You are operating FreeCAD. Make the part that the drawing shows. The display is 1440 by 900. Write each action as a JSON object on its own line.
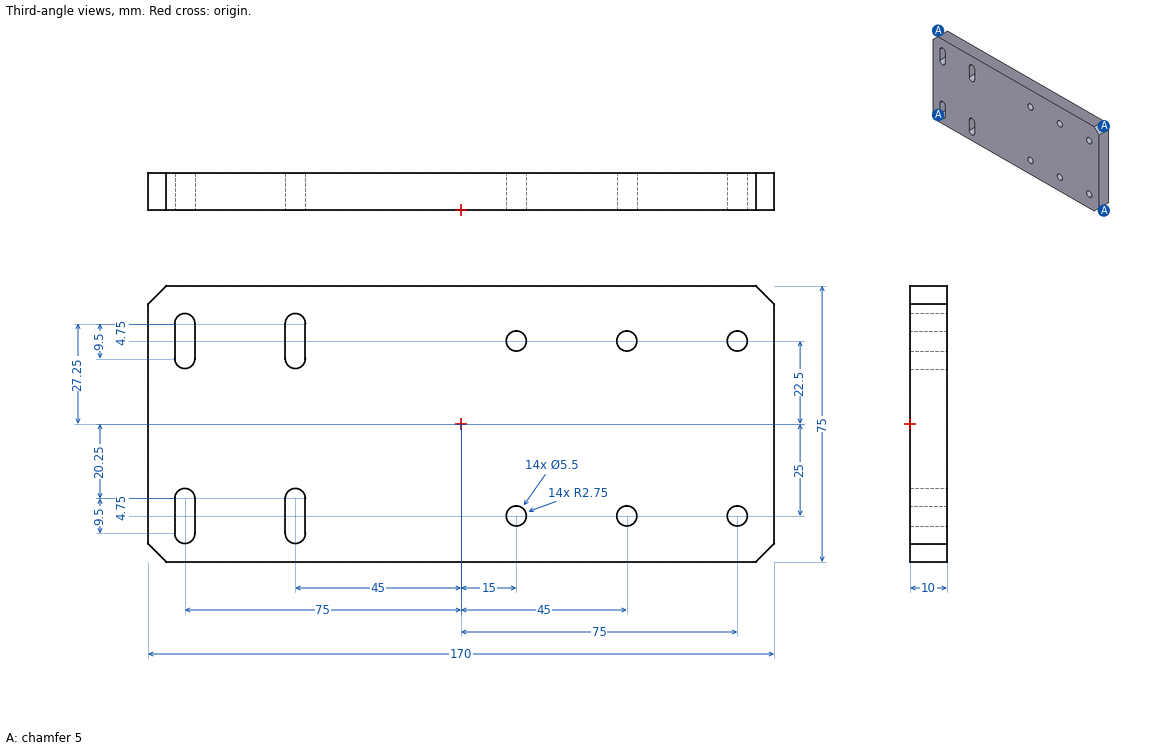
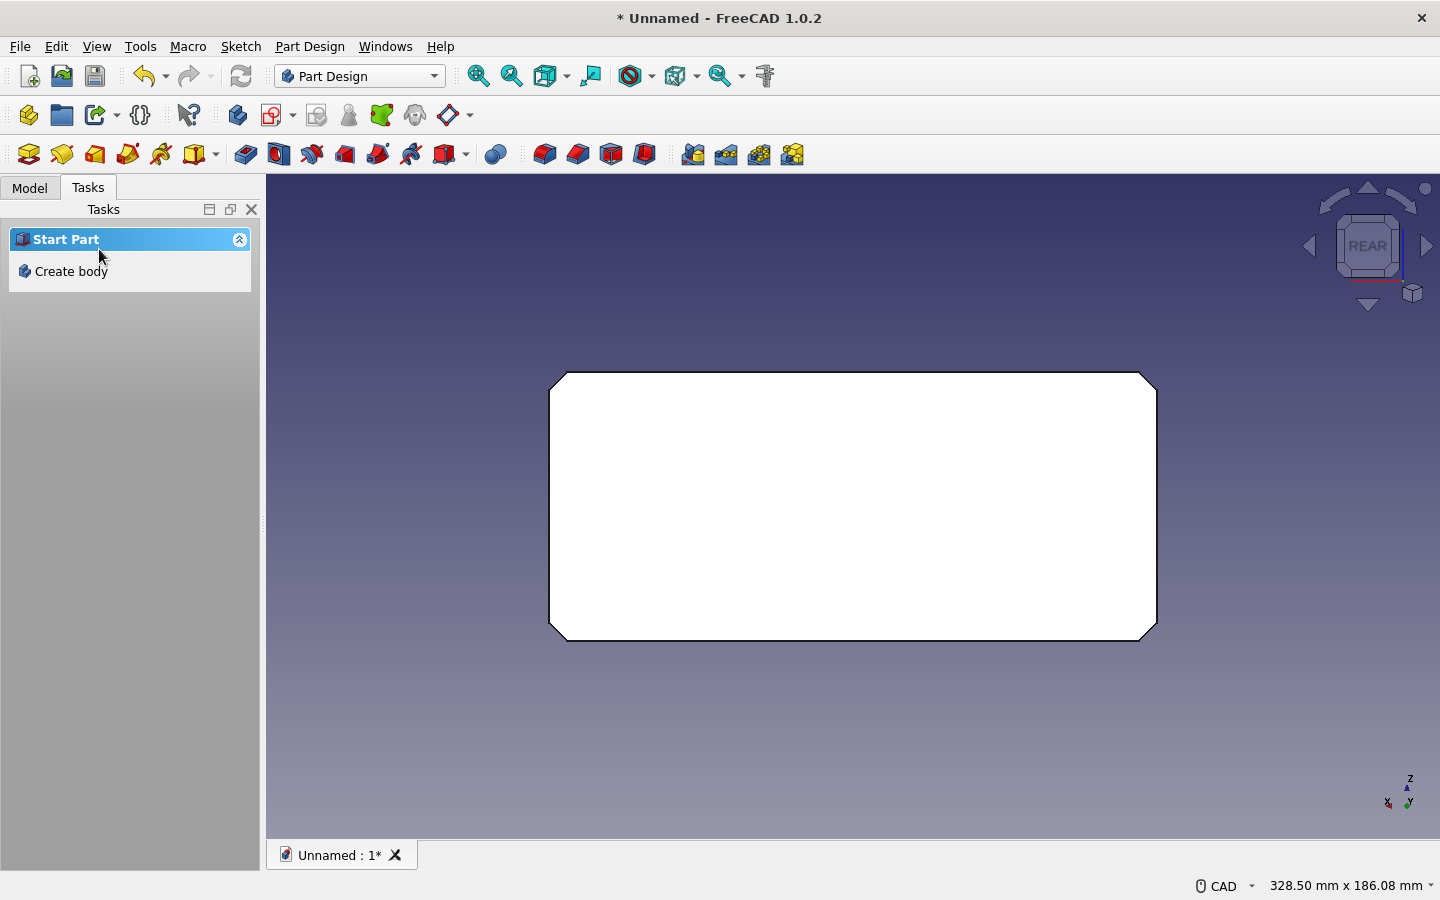
{"action": "left_click", "coordinate": [766, 506]}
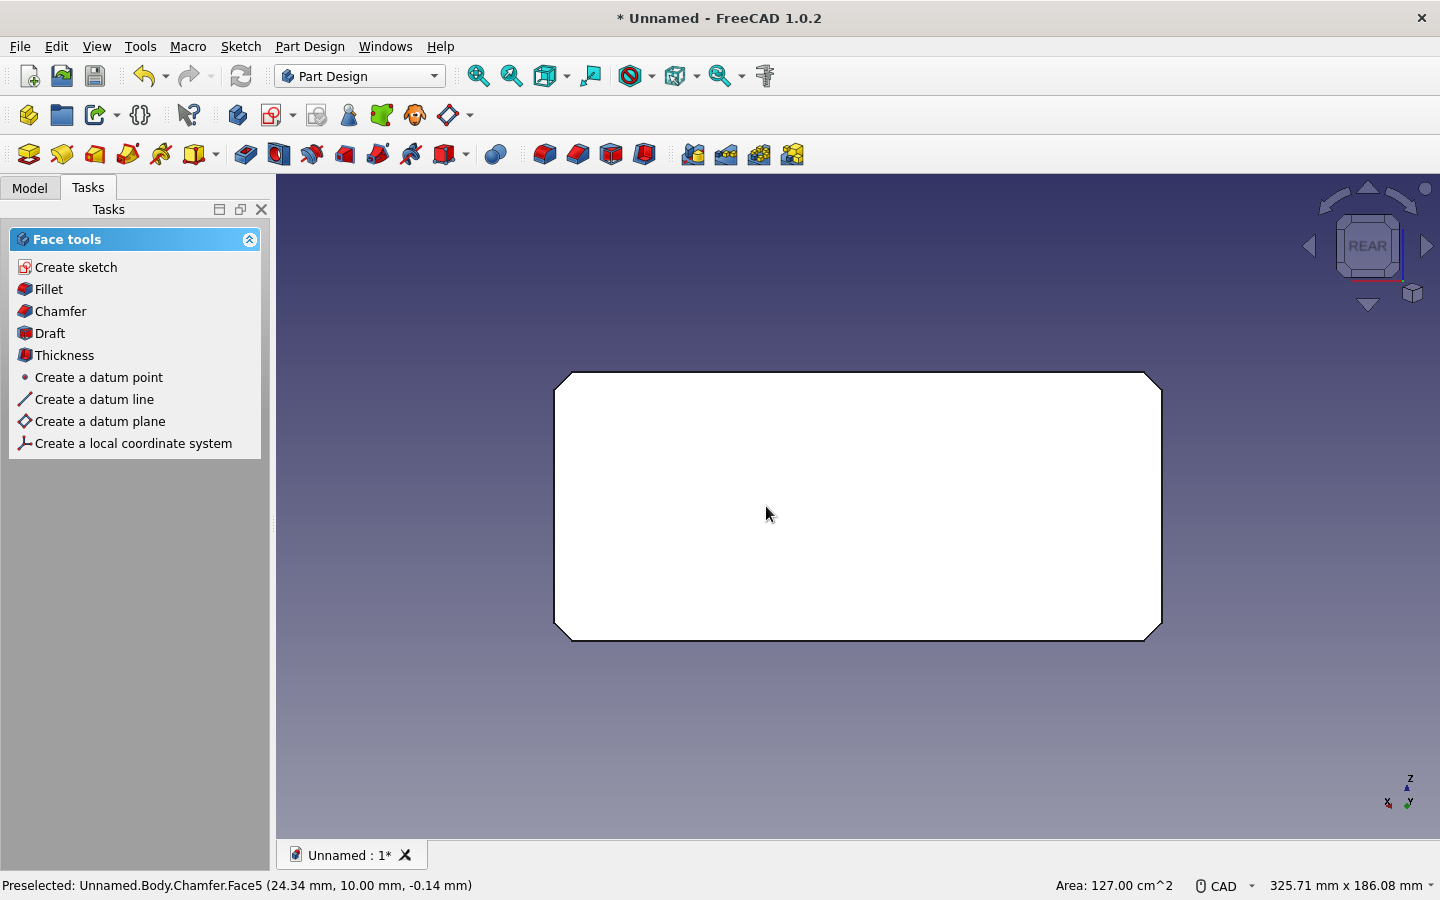
{"action": "left_click", "coordinate": [270, 116]}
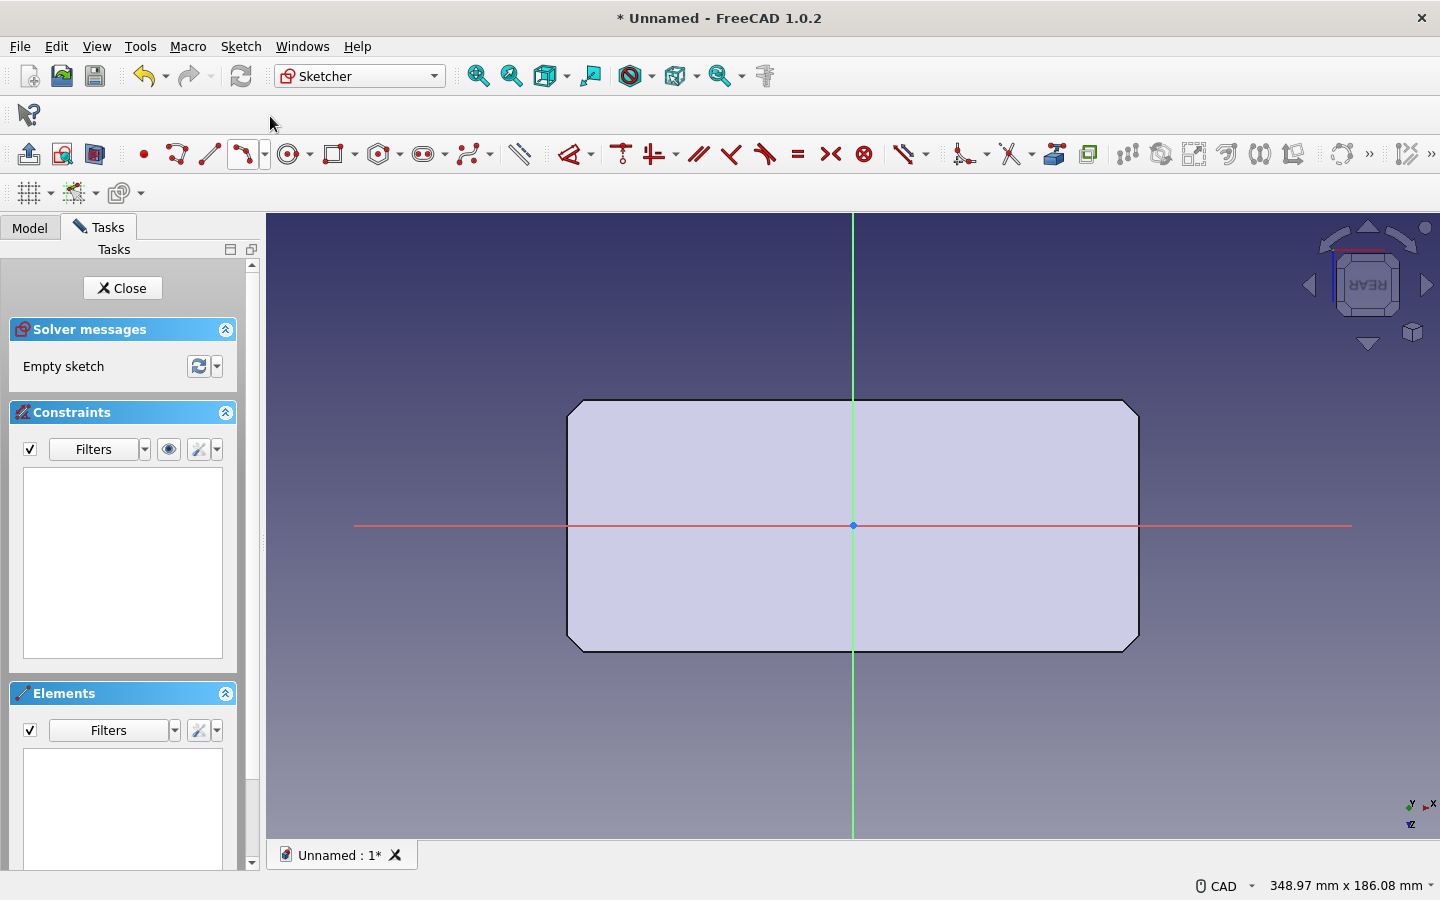
{"action": "key", "text": "g s"}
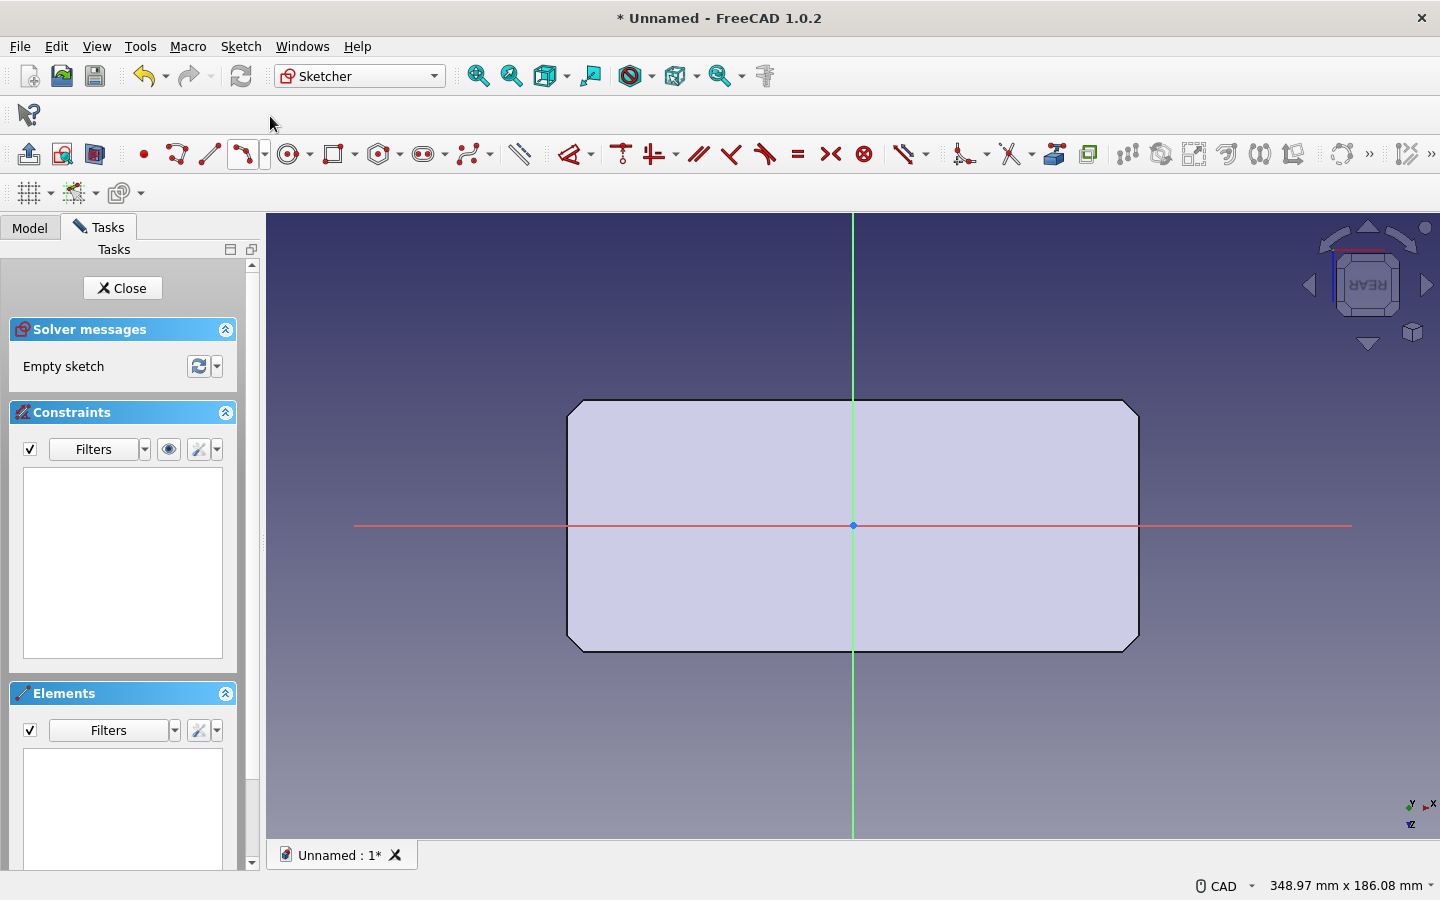
{"action": "scroll", "coordinate": [601, 458], "scroll_direction": "up", "scroll_amount": 5}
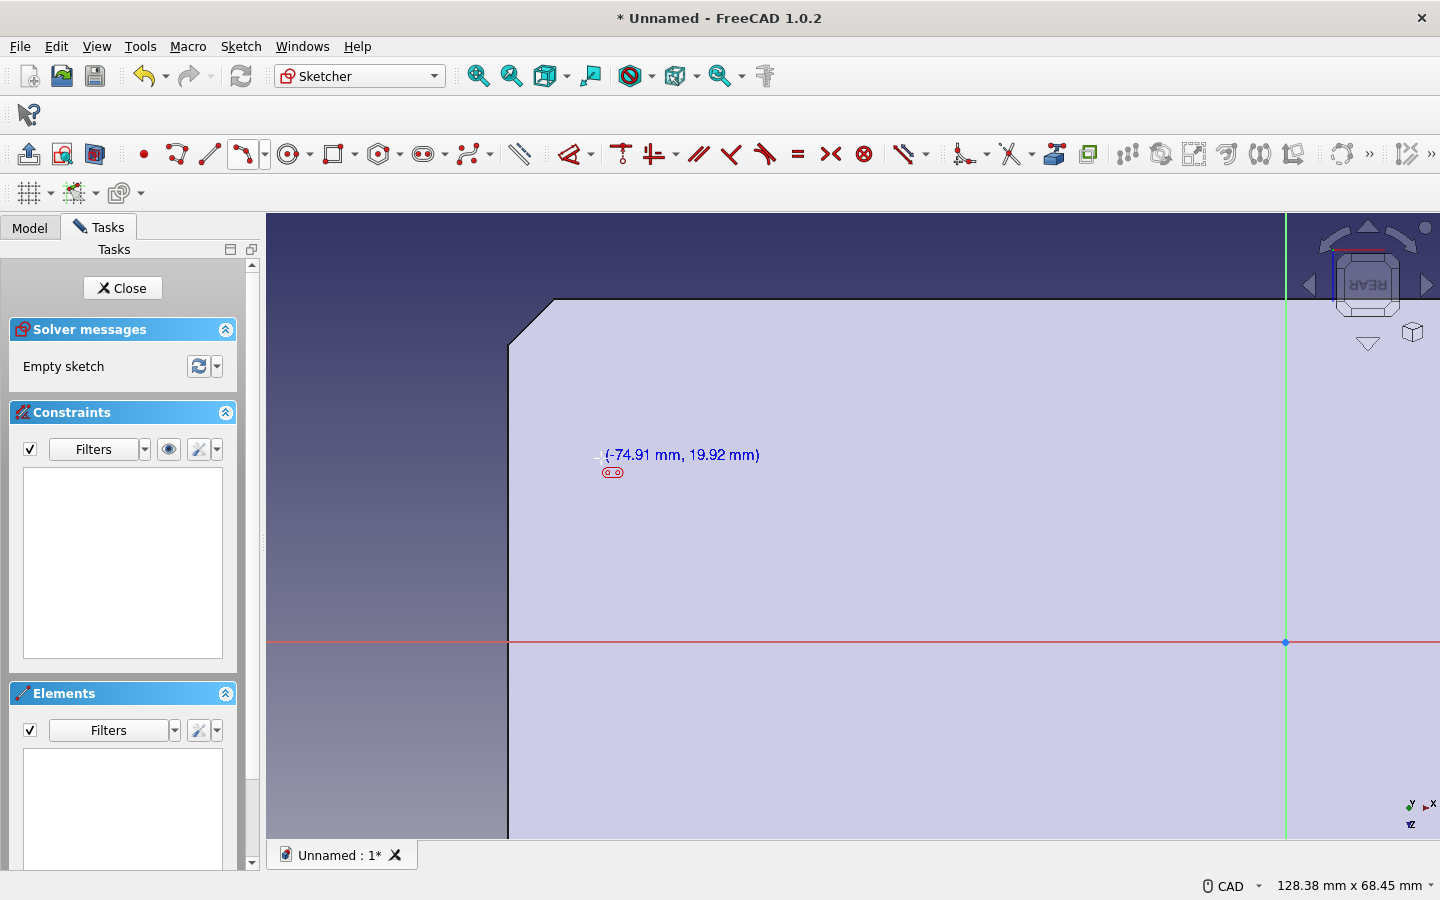
{"action": "left_click", "coordinate": [600, 457]}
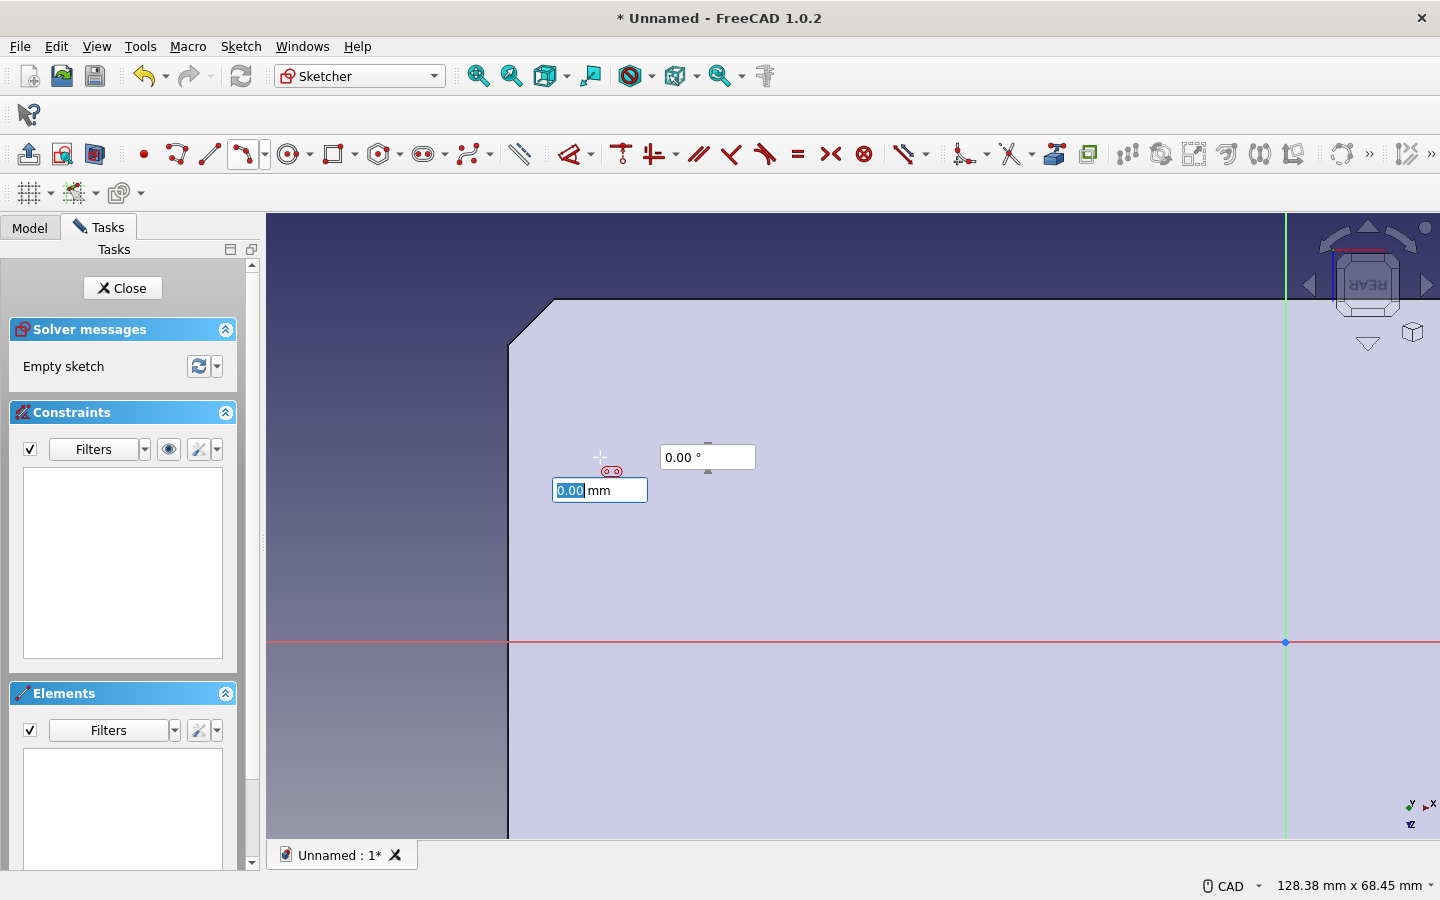
{"action": "left_click", "coordinate": [600, 370]}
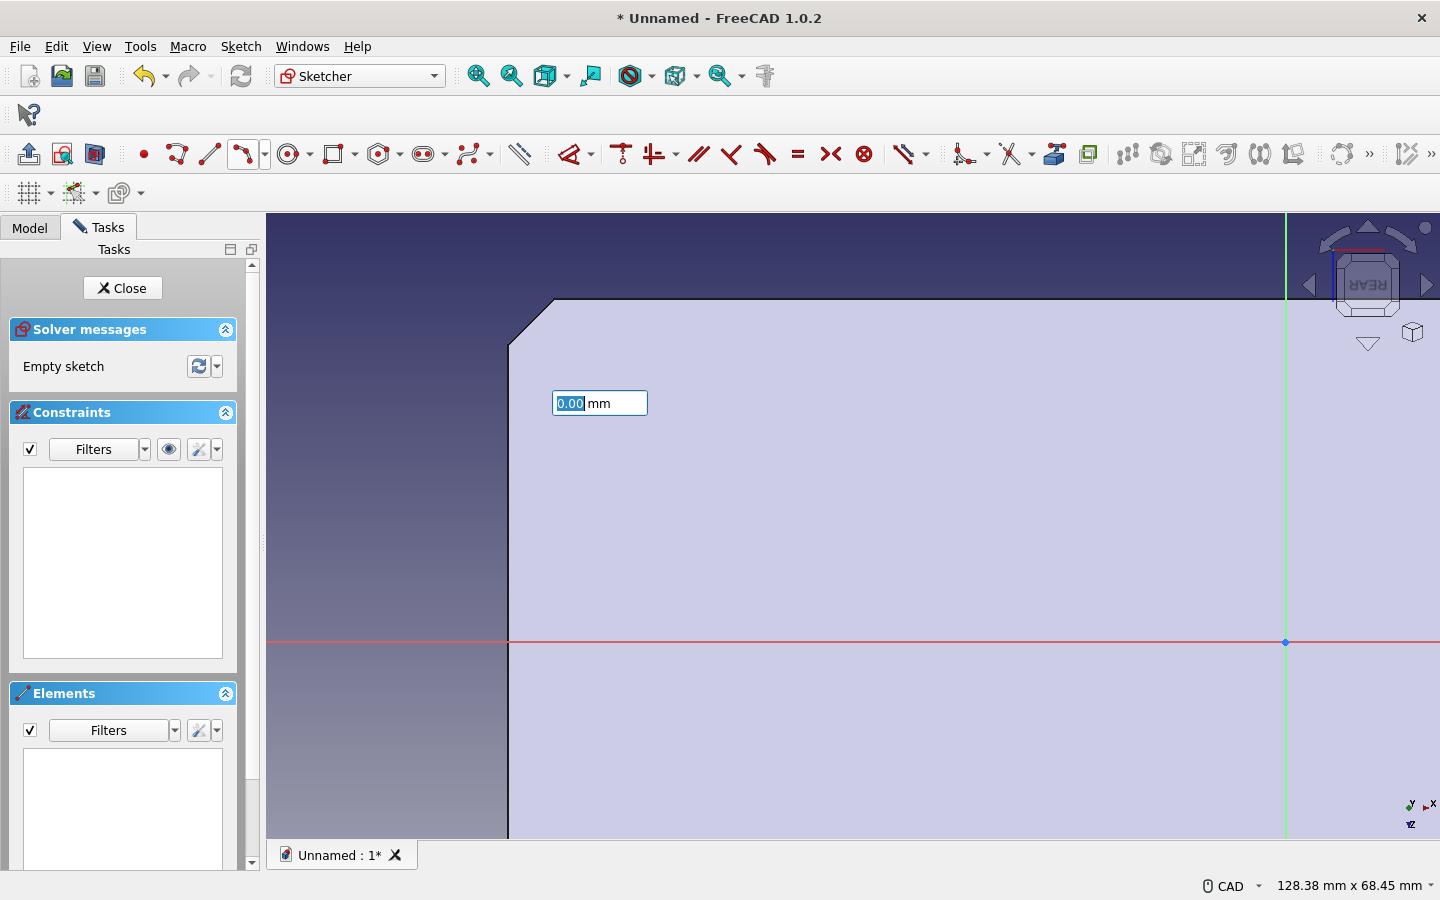
{"action": "left_click", "coordinate": [625, 414]}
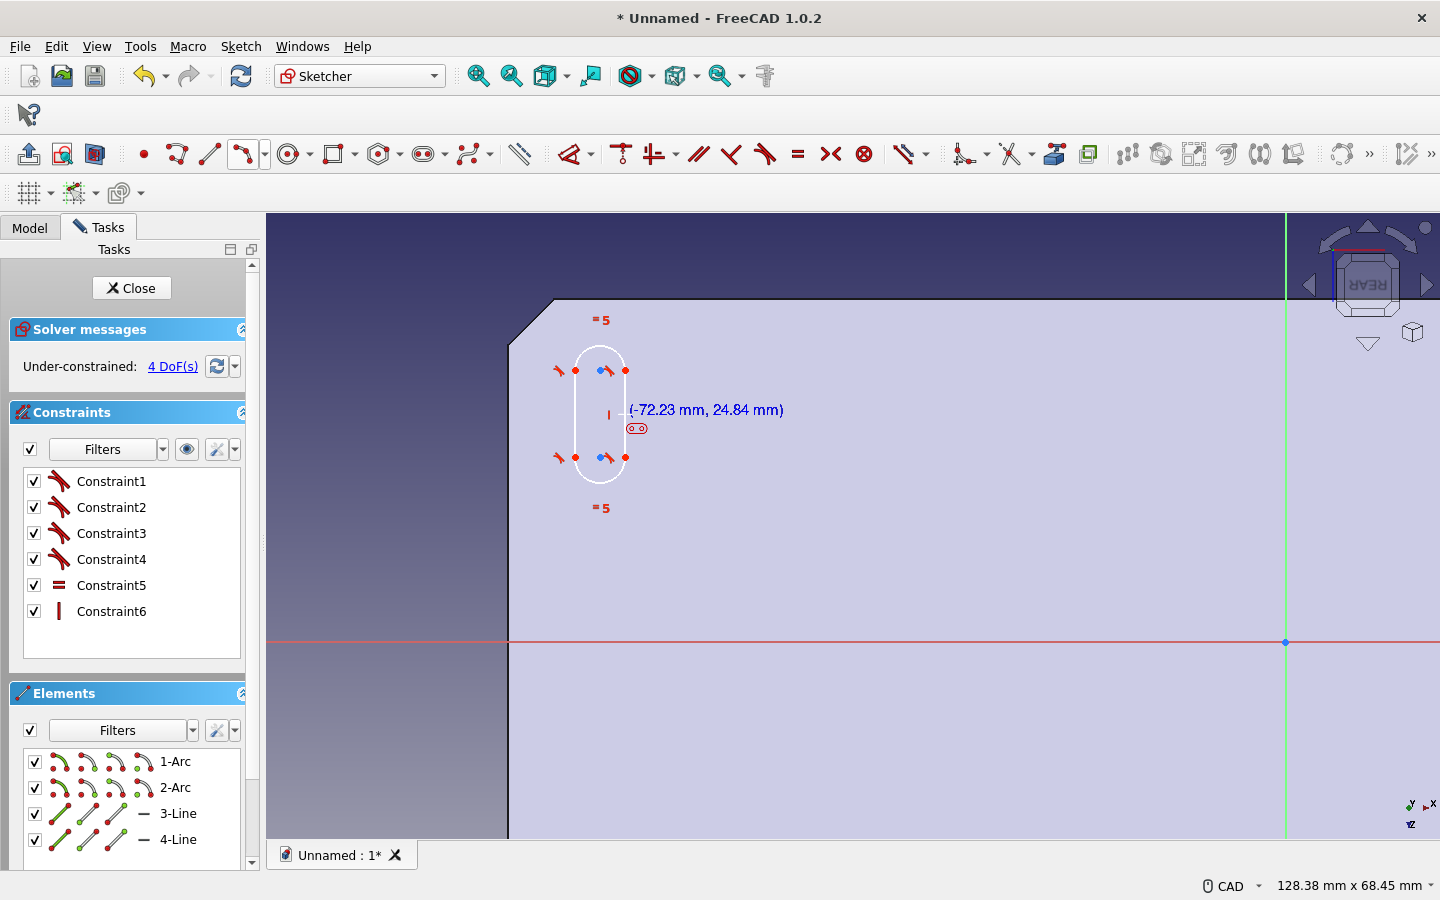
{"action": "left_click", "coordinate": [874, 457]}